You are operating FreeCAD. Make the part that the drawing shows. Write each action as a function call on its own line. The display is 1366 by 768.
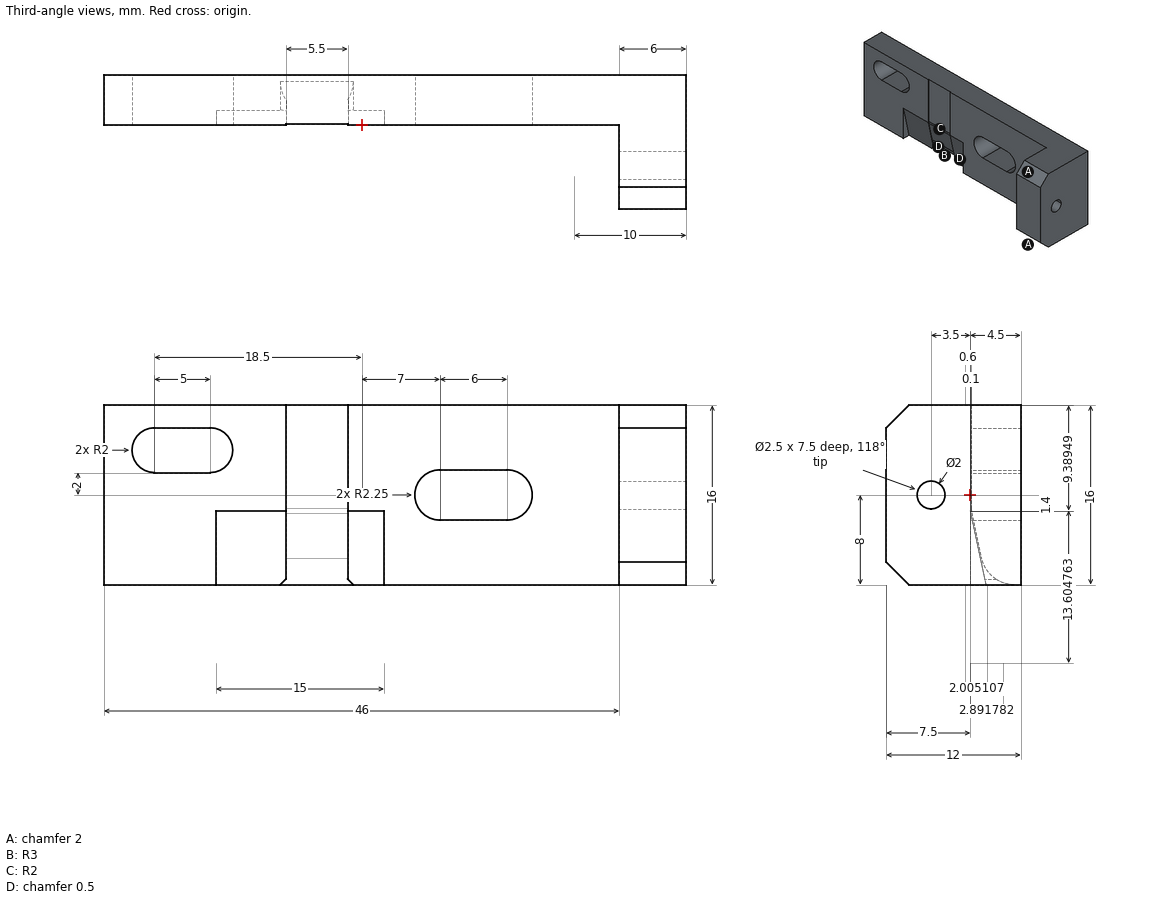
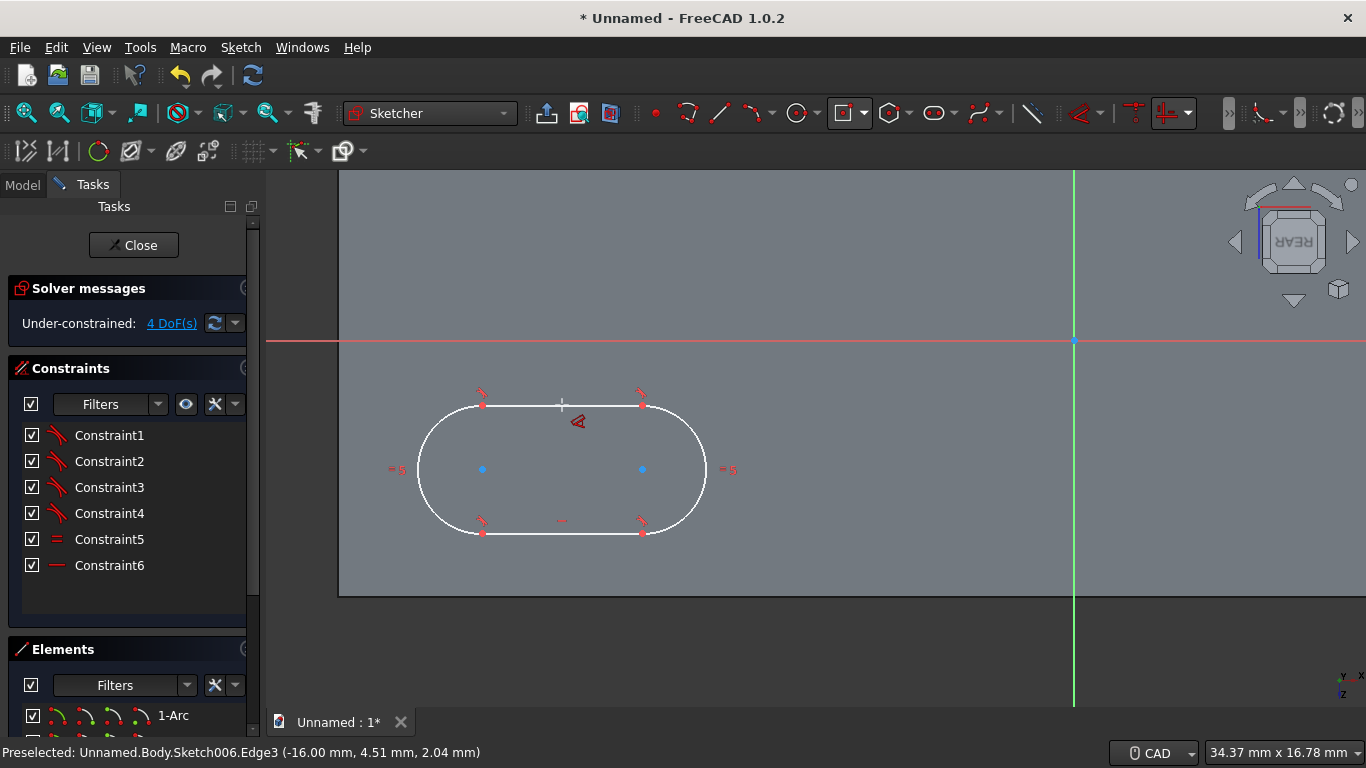
click(430, 432)
click(404, 413)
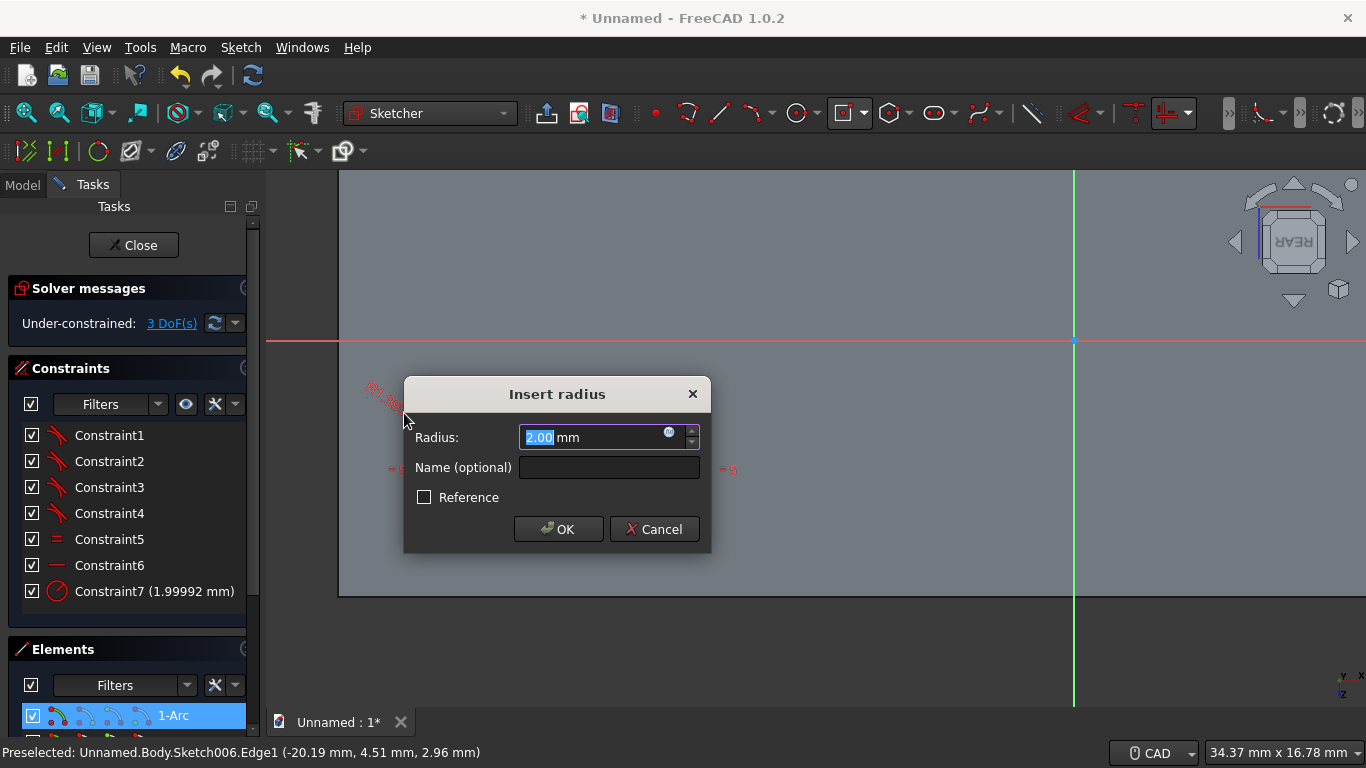
text(2)
key(Return)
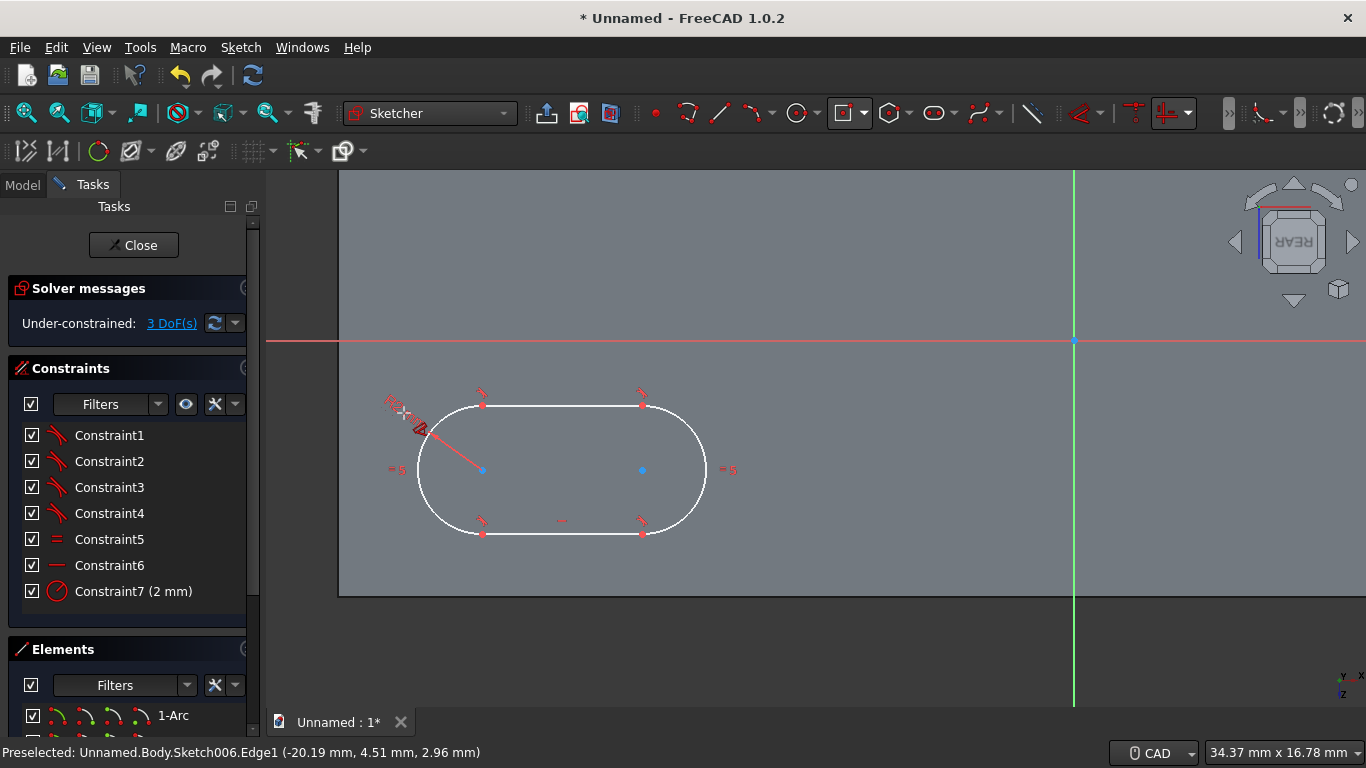
click(530, 406)
click(562, 372)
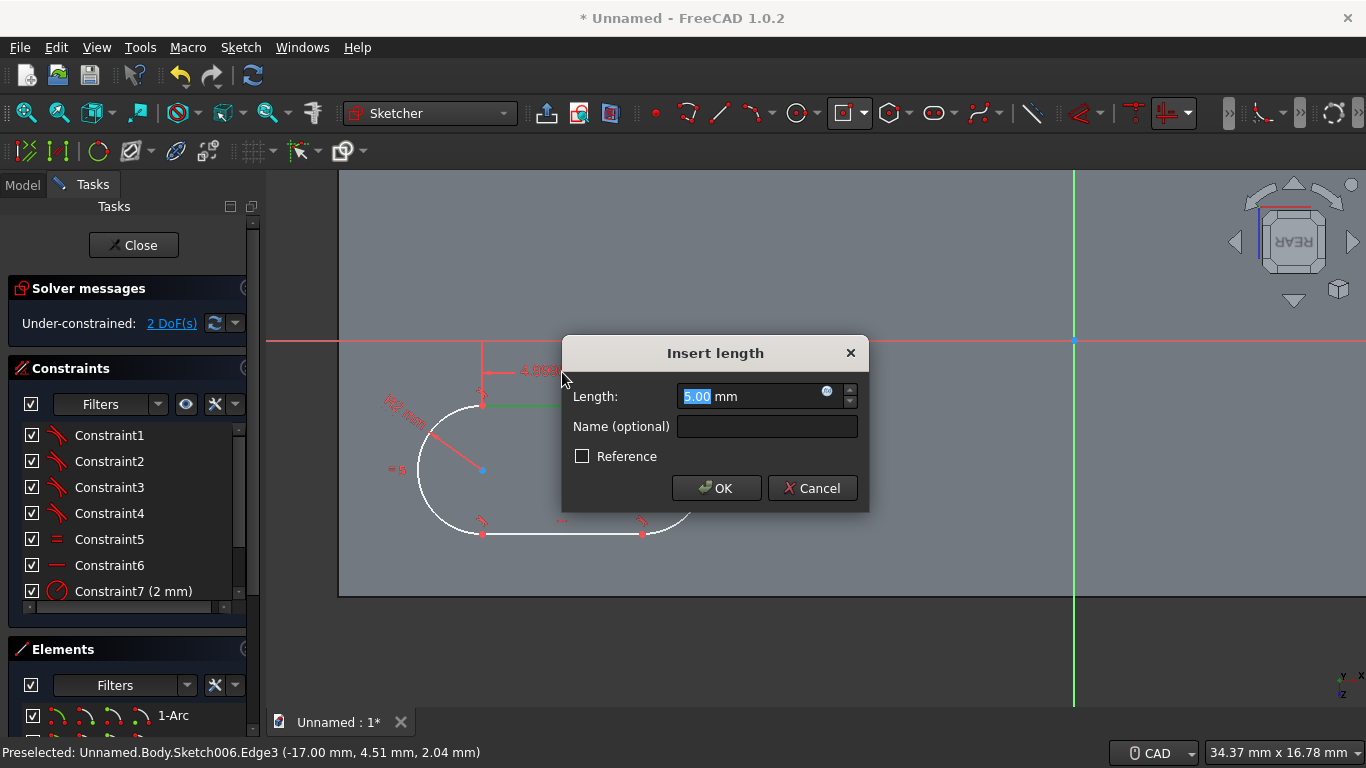
text(5)
key(Return)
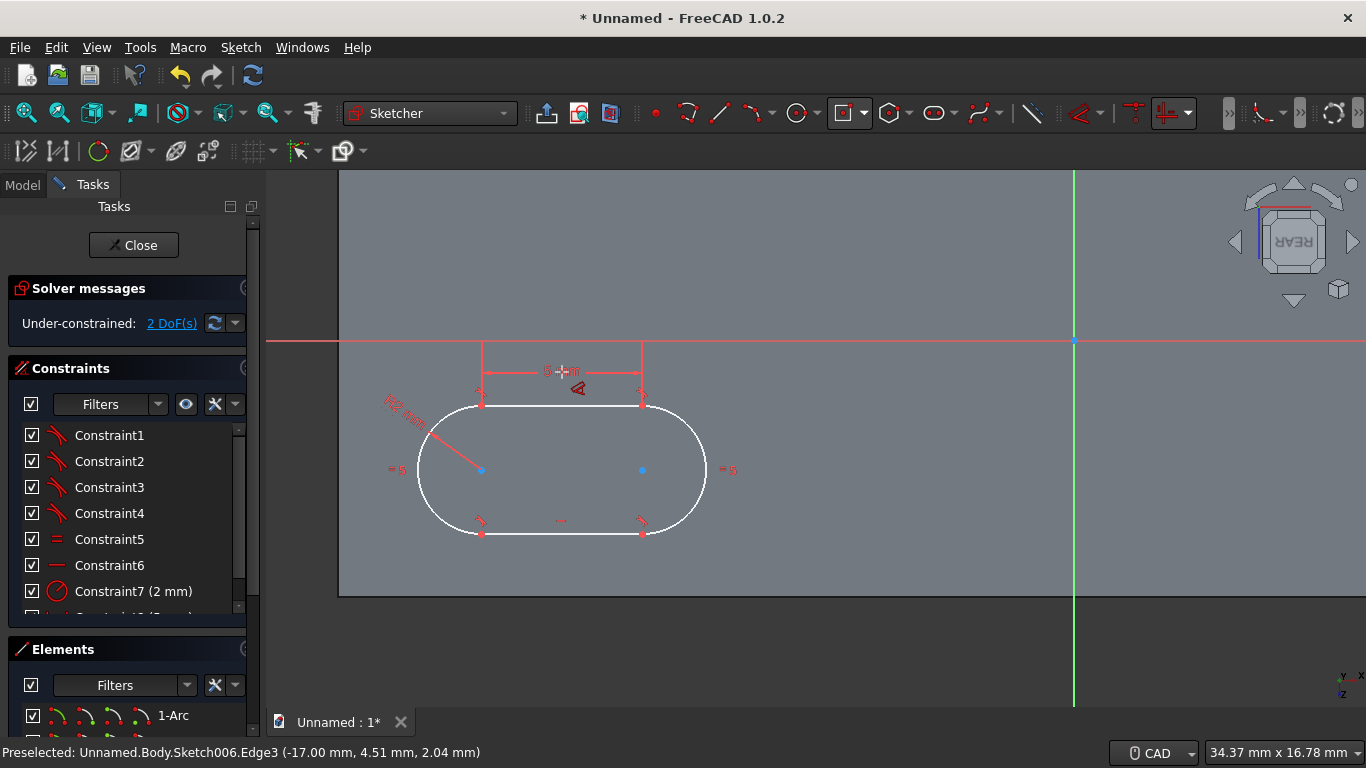
click(482, 406)
click(1108, 373)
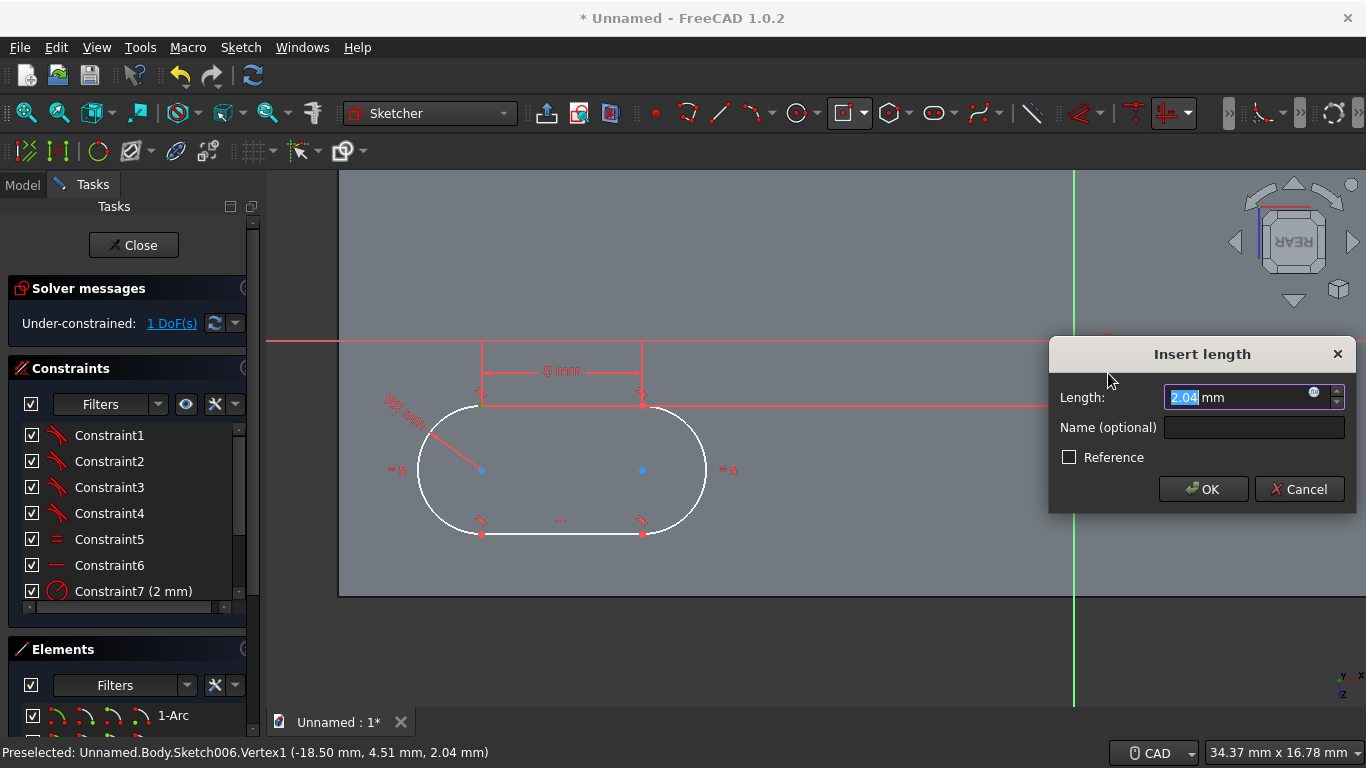
text(2)
key(Return)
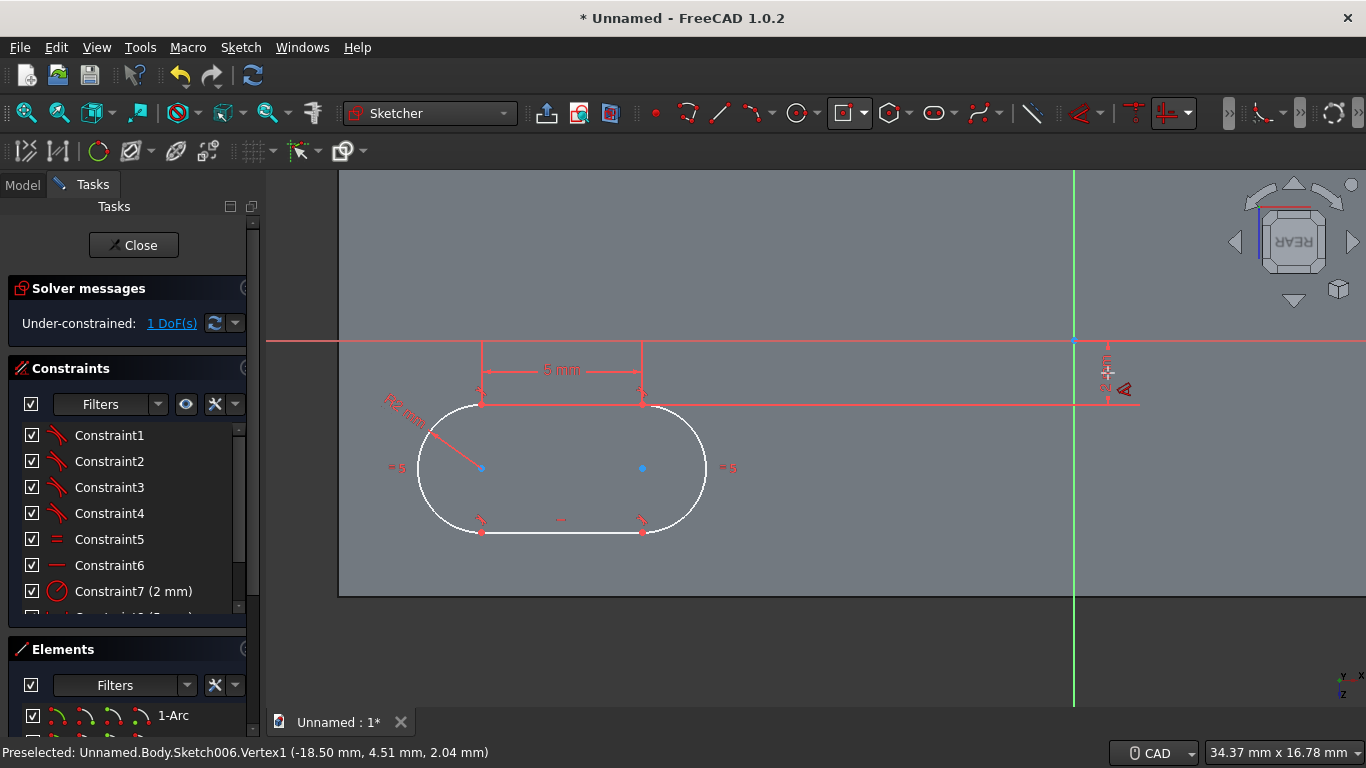
click(482, 405)
click(778, 307)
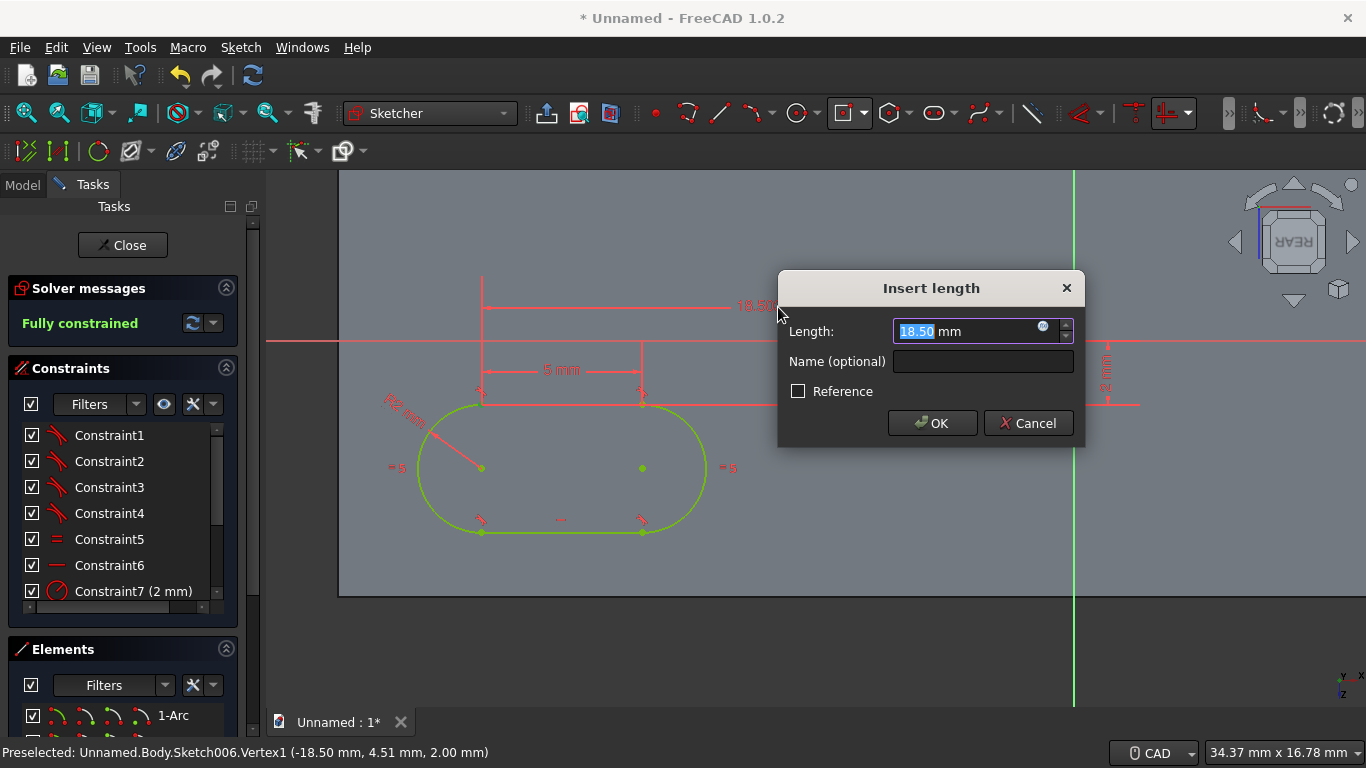
text(18.5)
key(Return)
key(Escape)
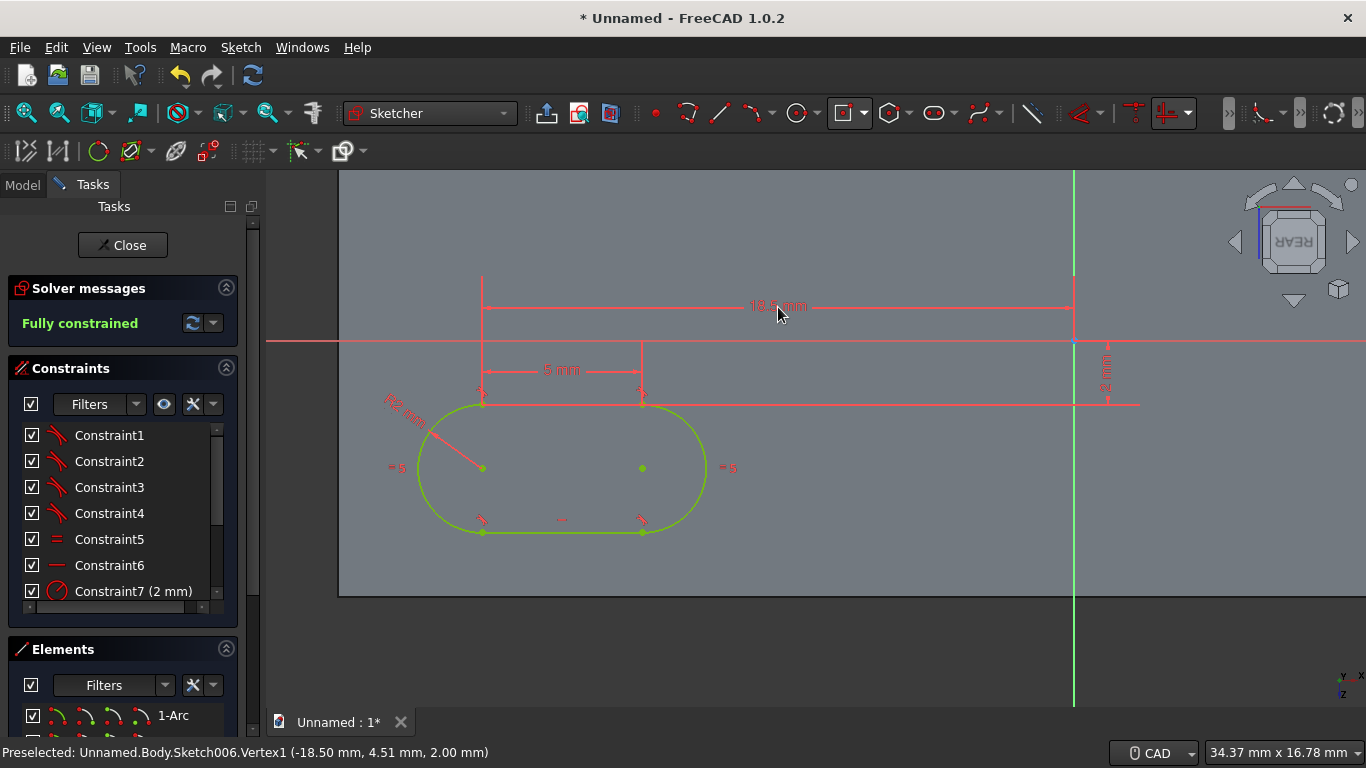
click(123, 245)